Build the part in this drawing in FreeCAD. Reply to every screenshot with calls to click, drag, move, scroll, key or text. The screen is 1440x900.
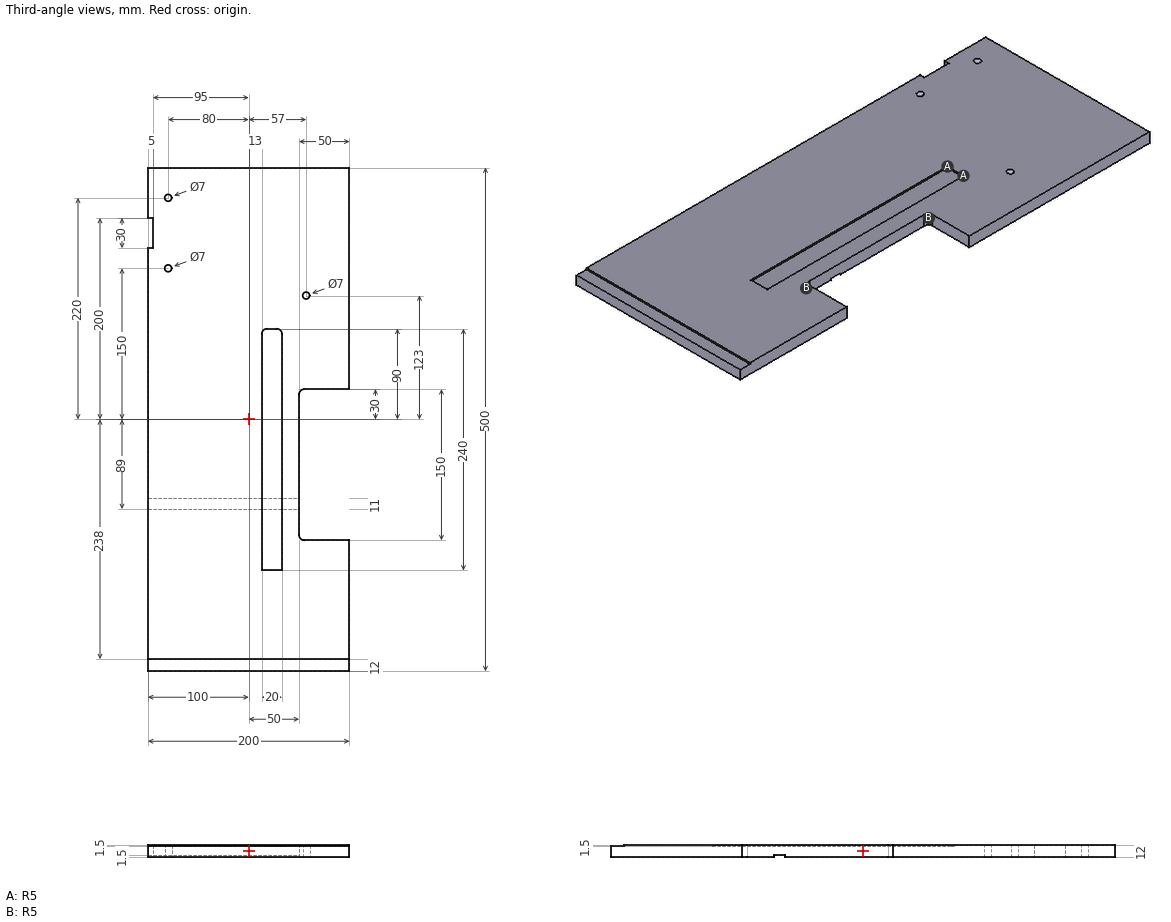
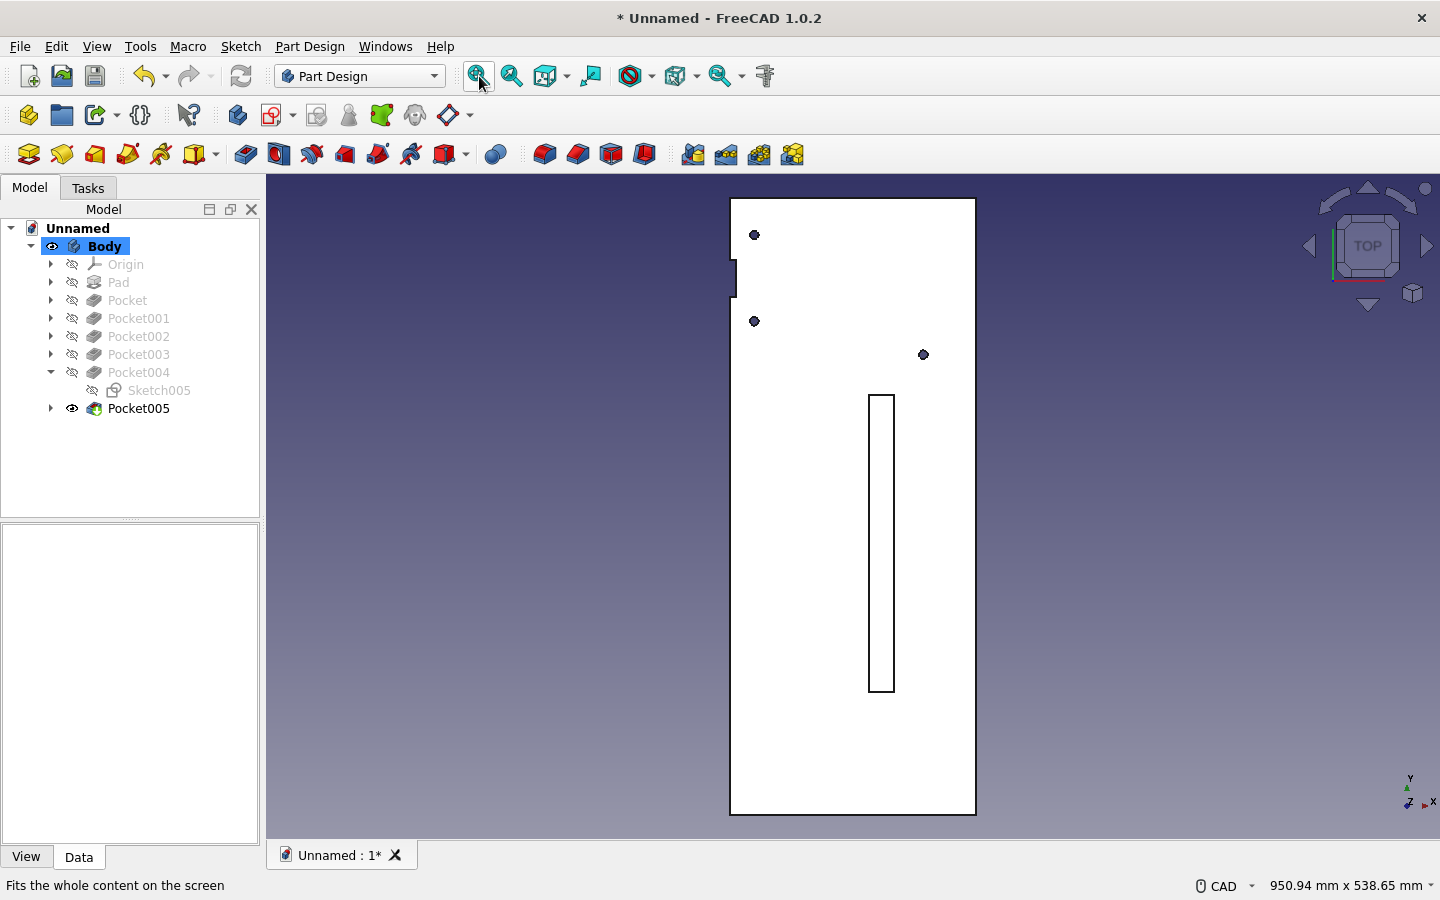
scroll(894, 394, up, 15)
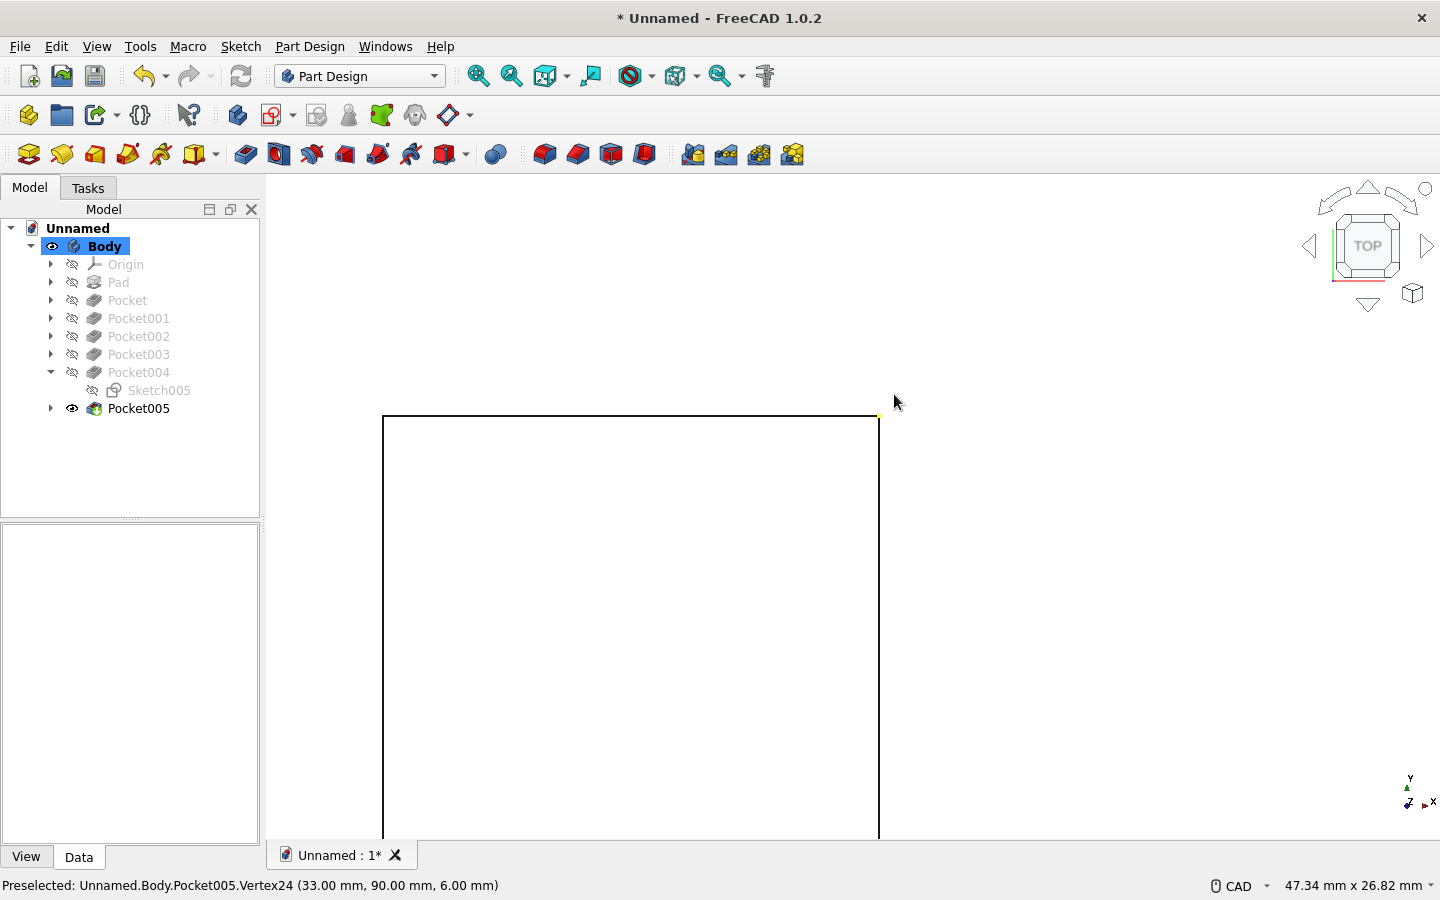
key(v)
key(f)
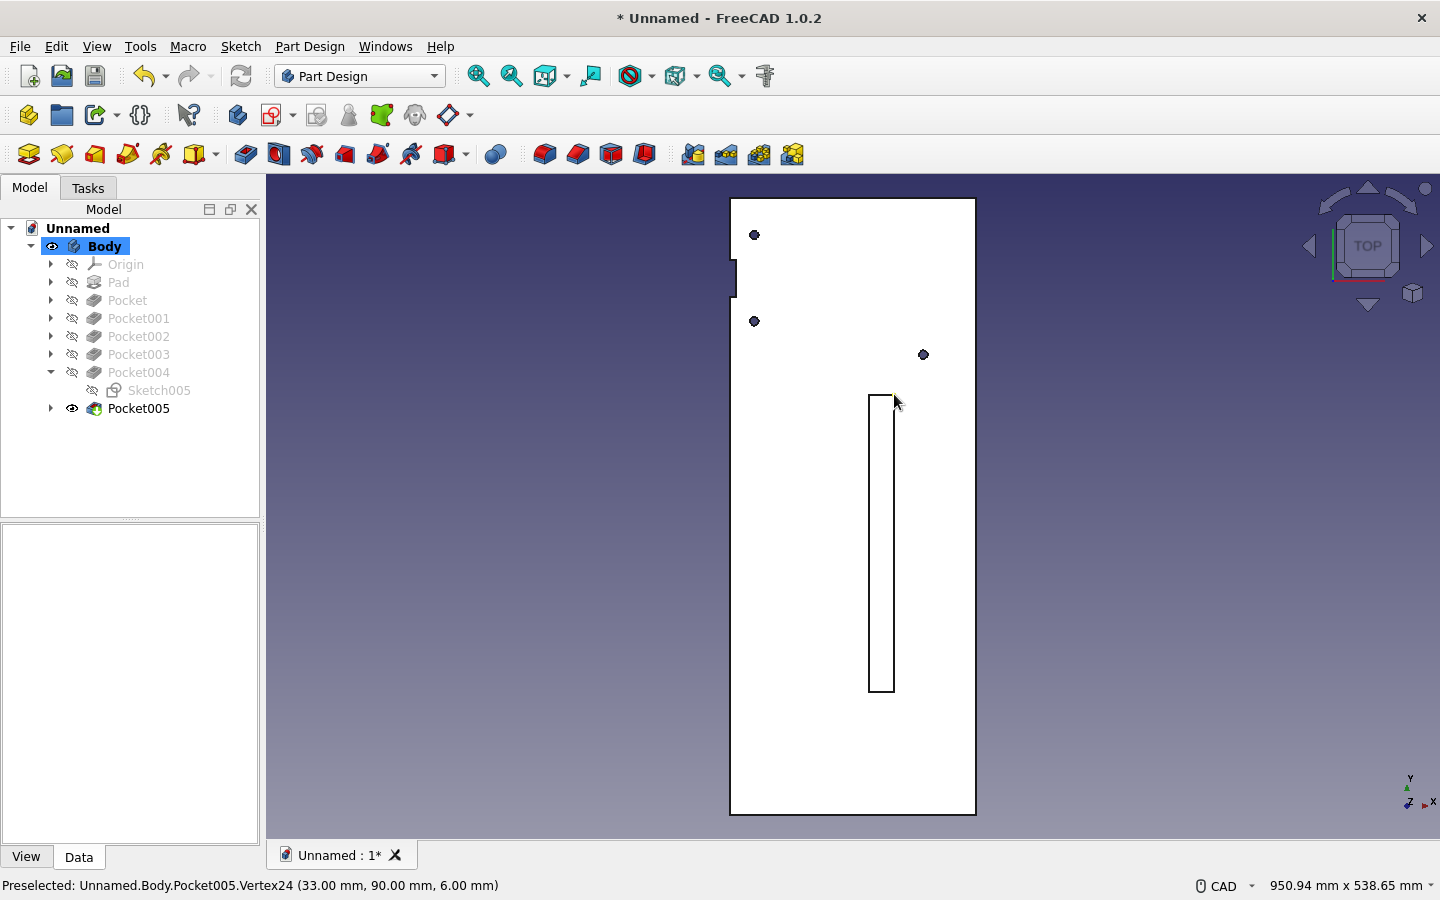
key(0)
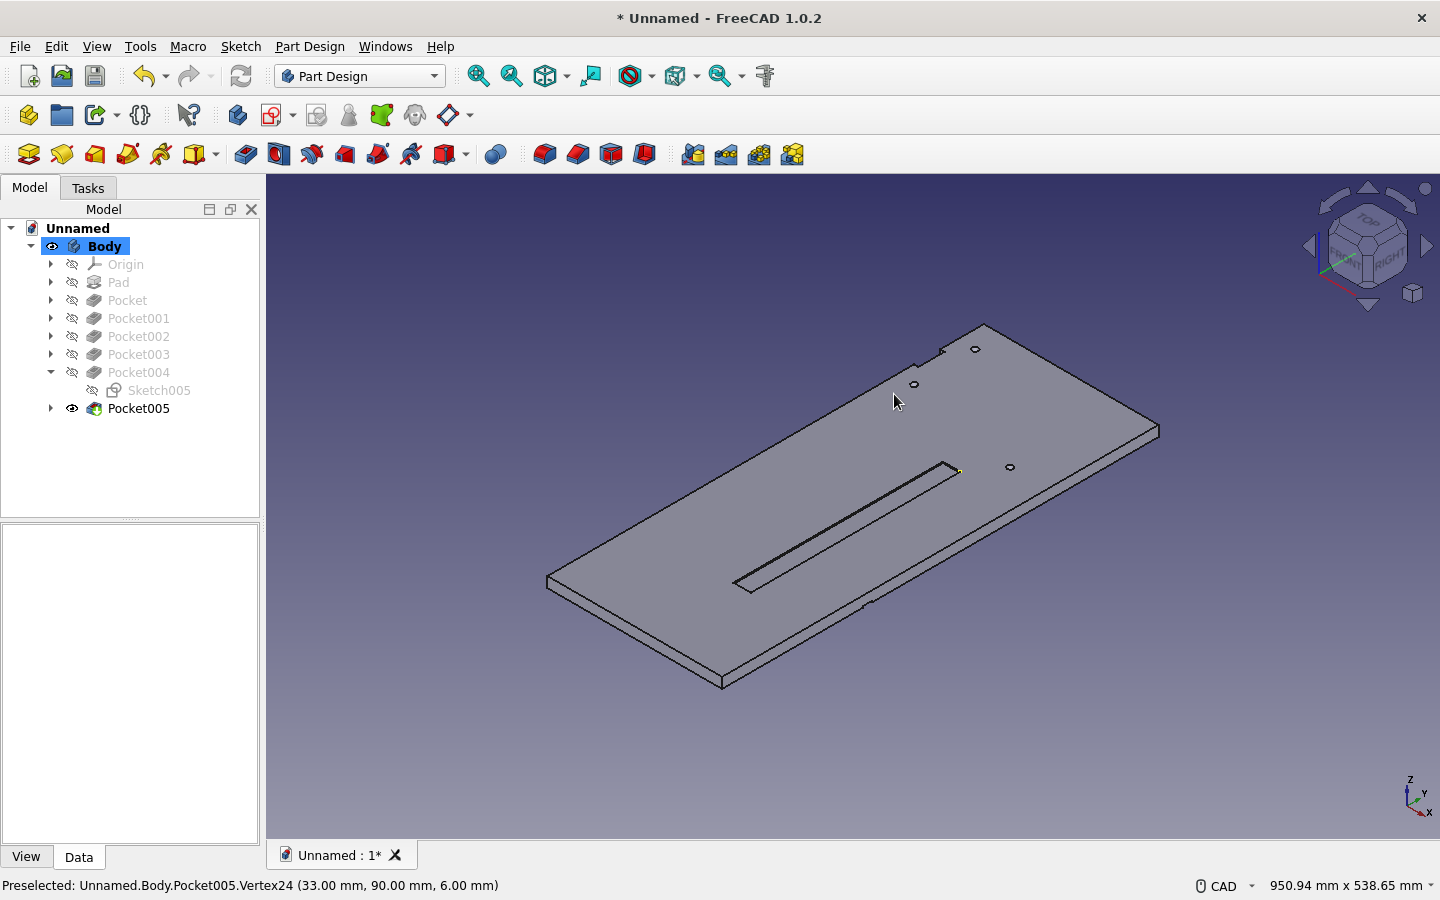
scroll(960, 471, up, 15)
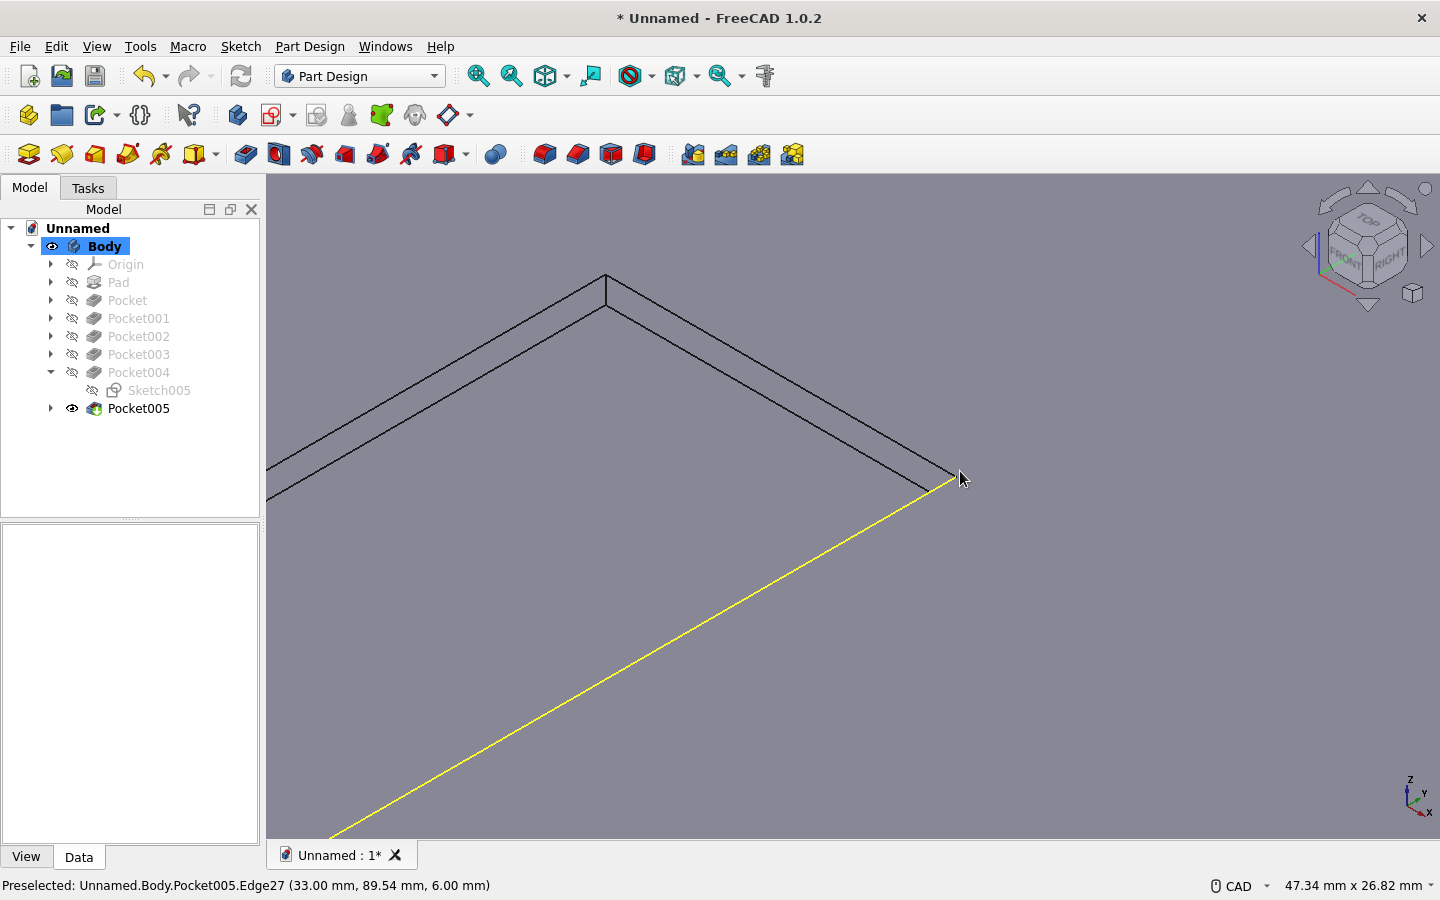
click(479, 76)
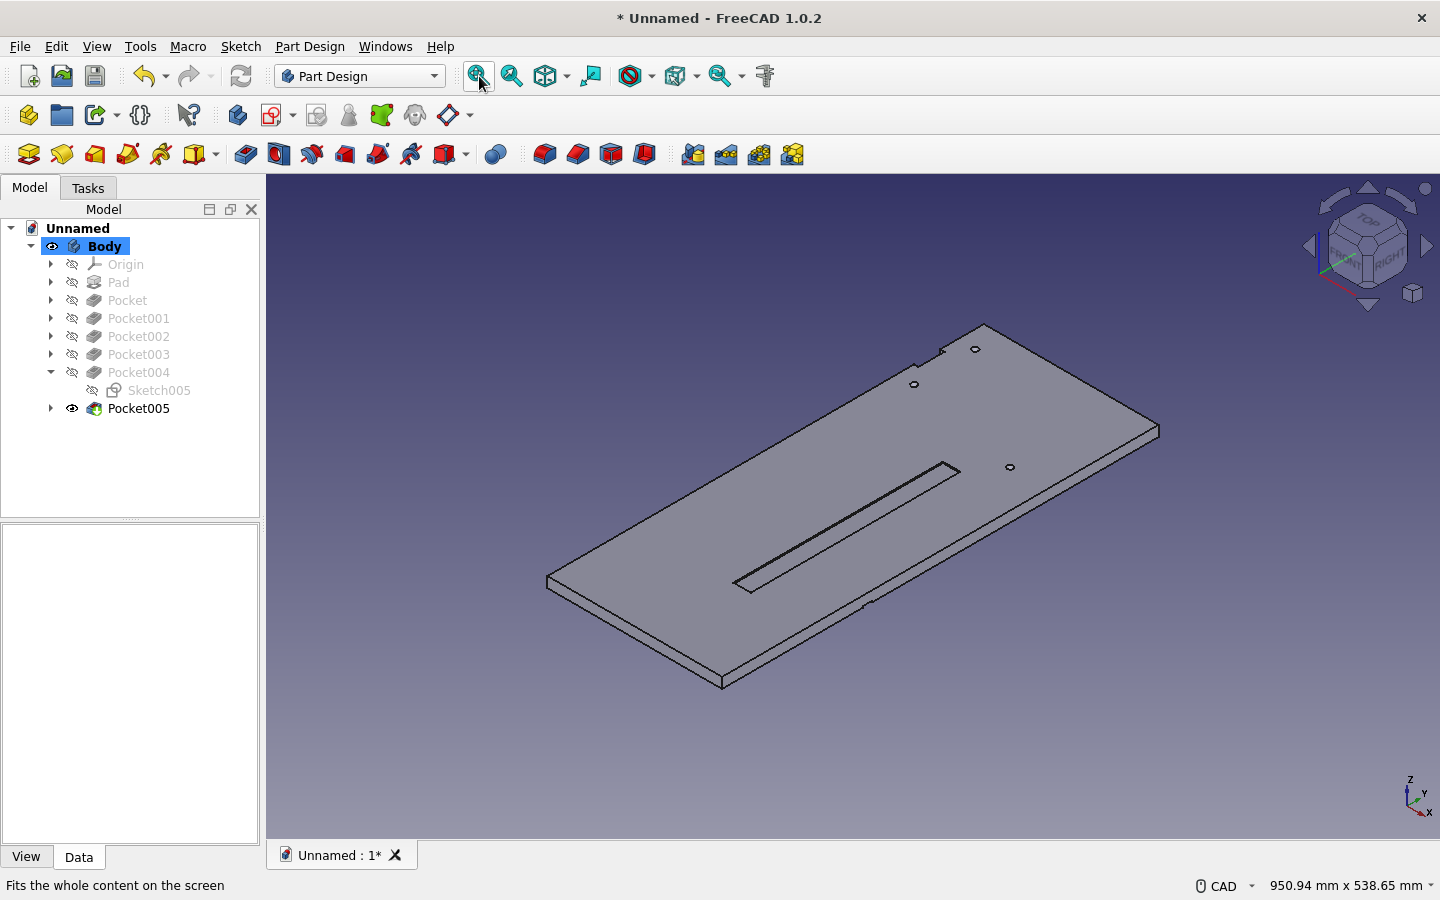
key(1)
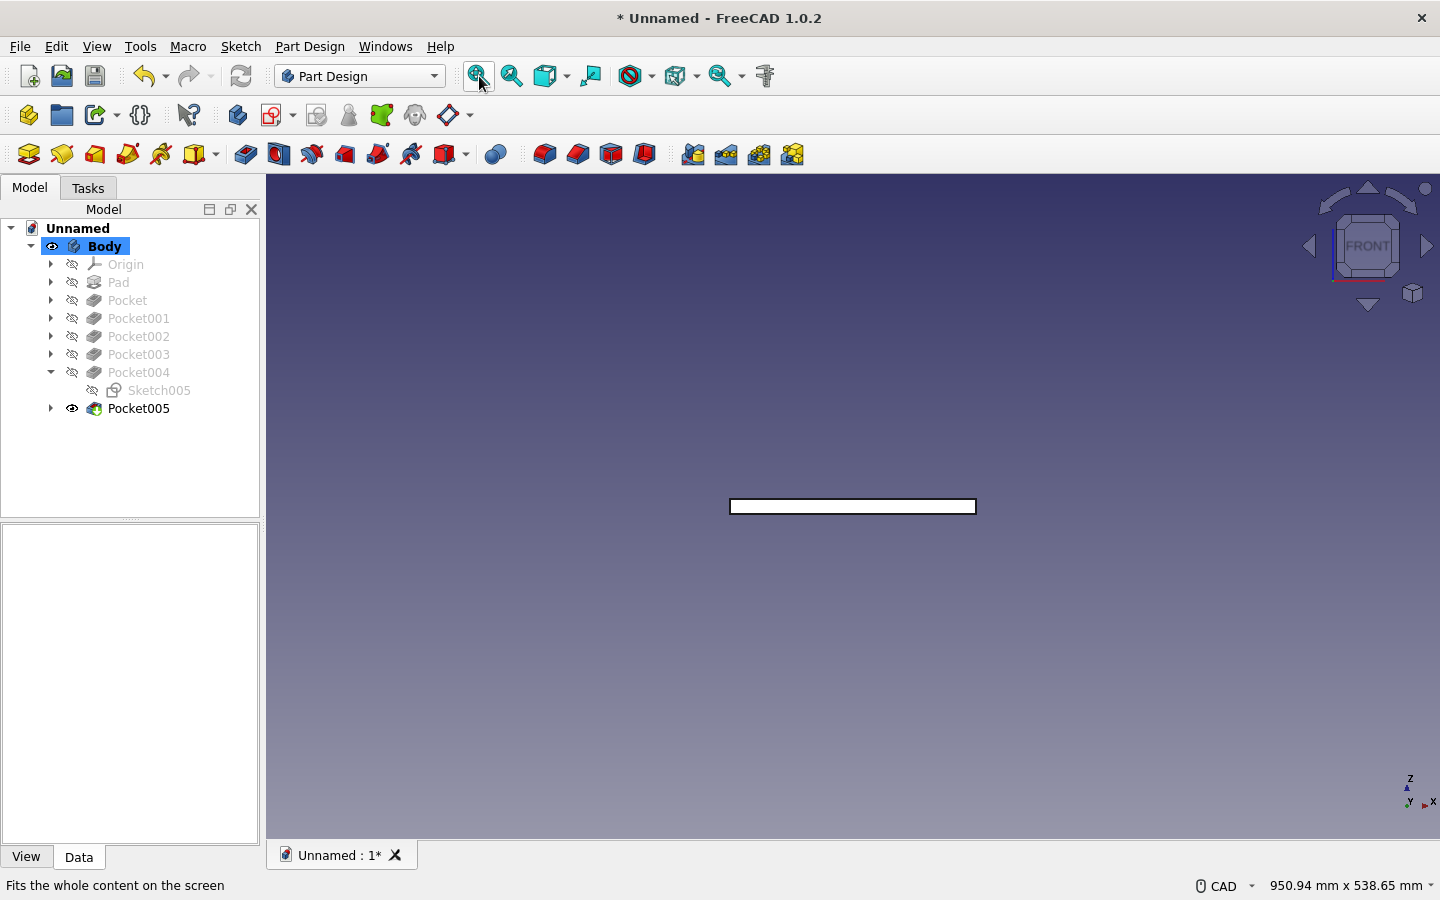
click(479, 76)